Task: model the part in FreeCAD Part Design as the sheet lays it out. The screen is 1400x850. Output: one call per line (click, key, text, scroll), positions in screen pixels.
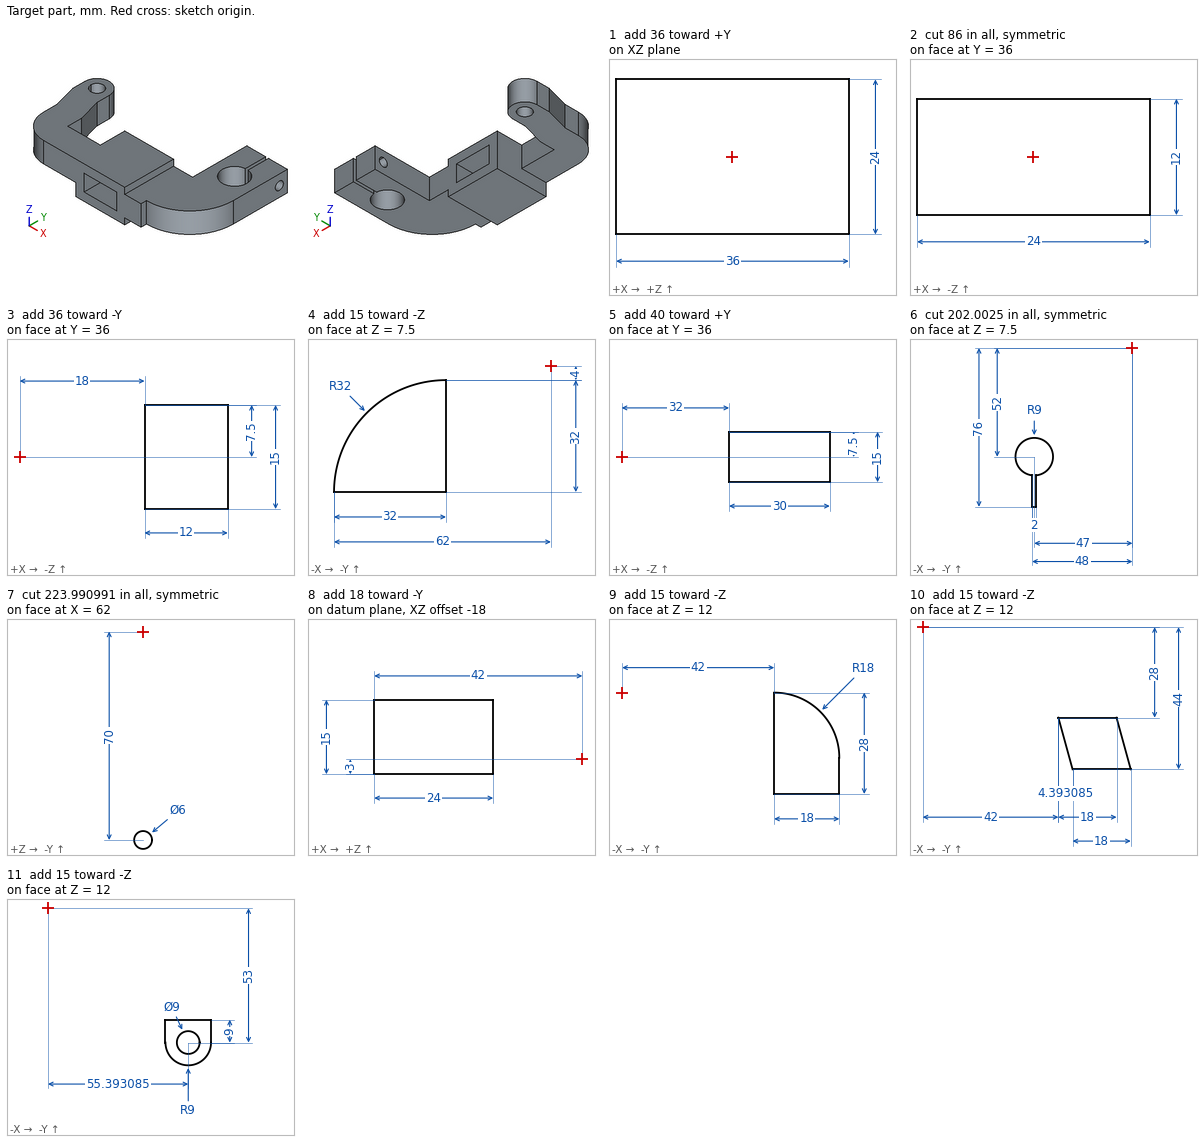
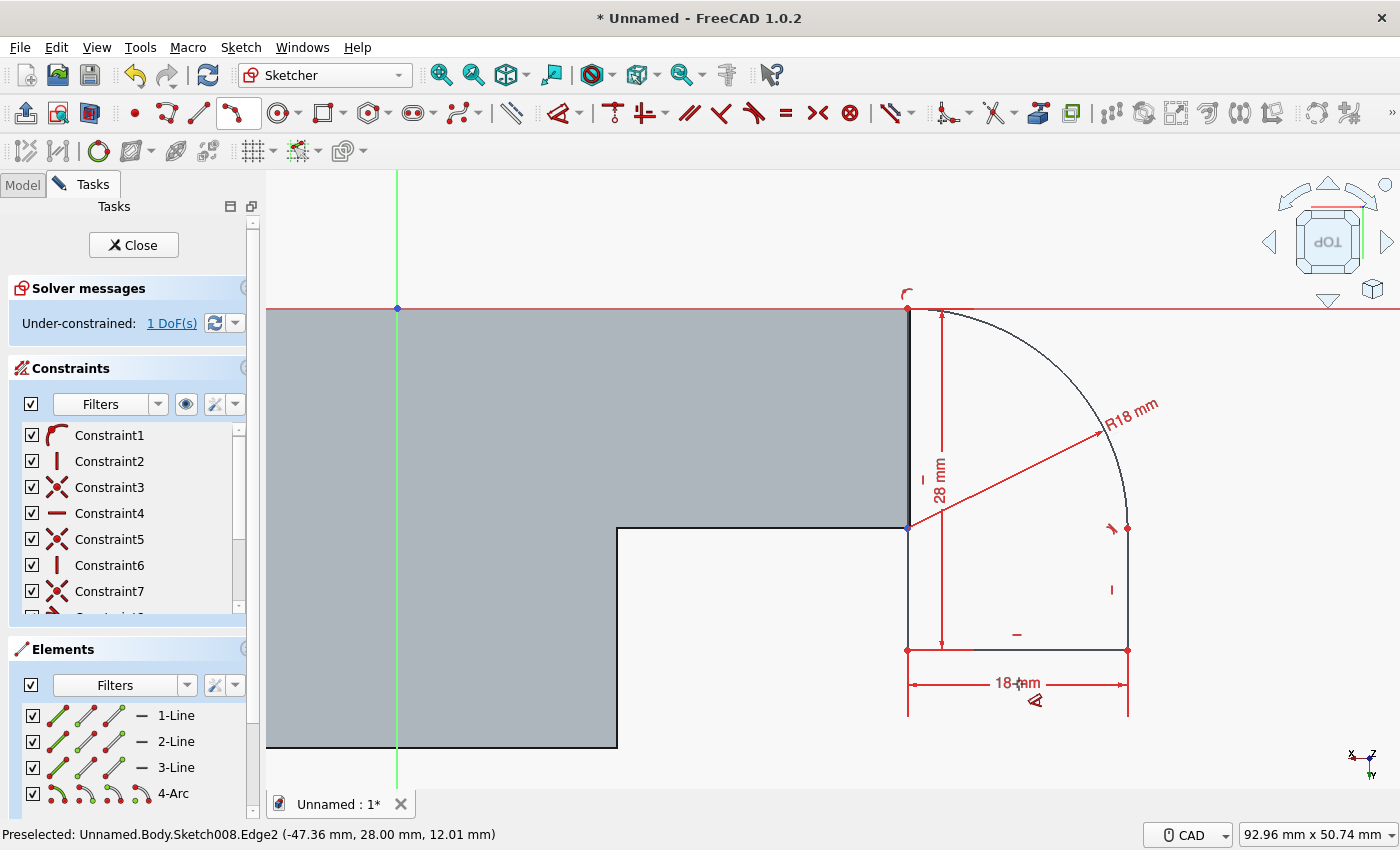
click(908, 309)
click(653, 275)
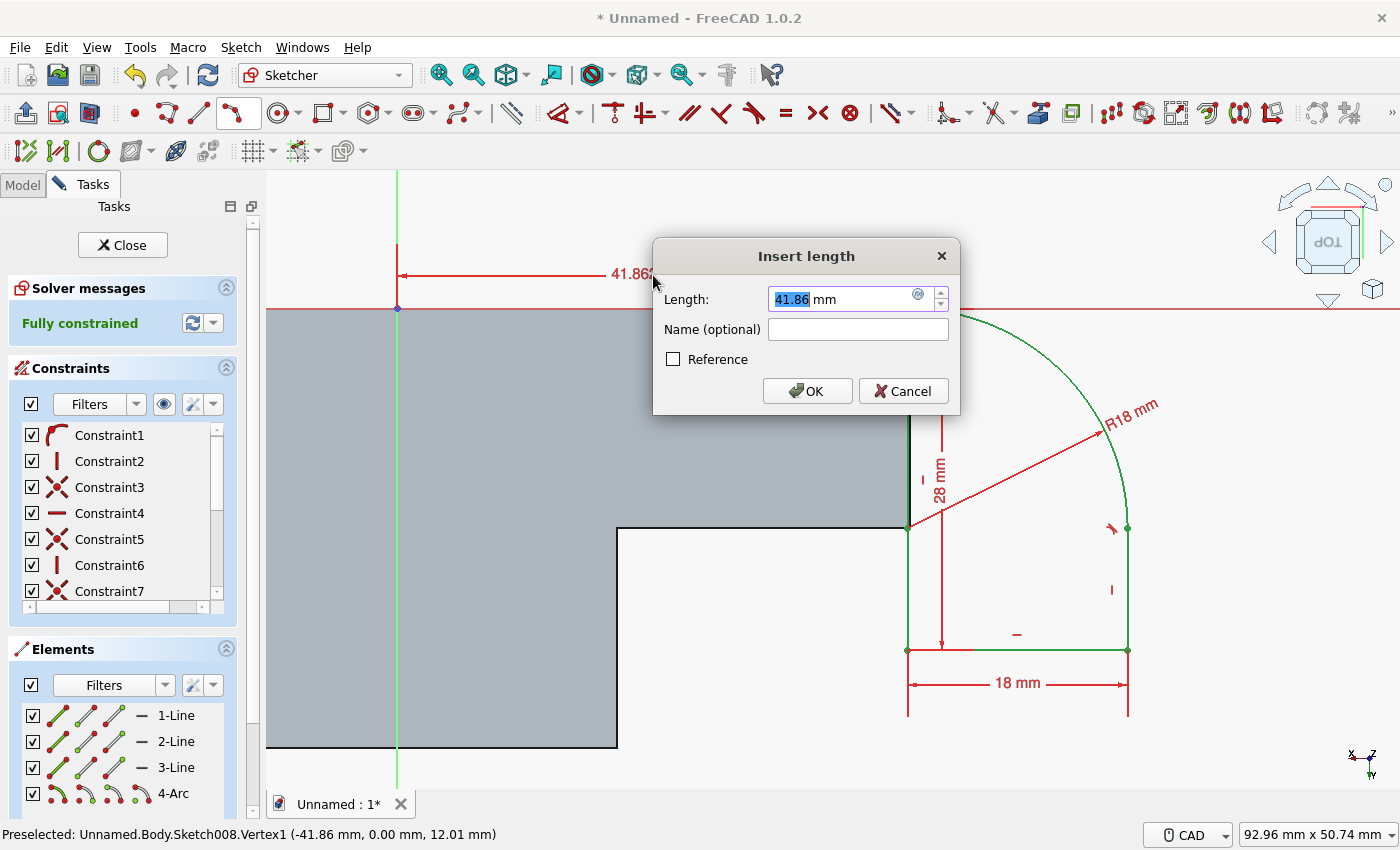
text(42)
key(Return)
key(Escape)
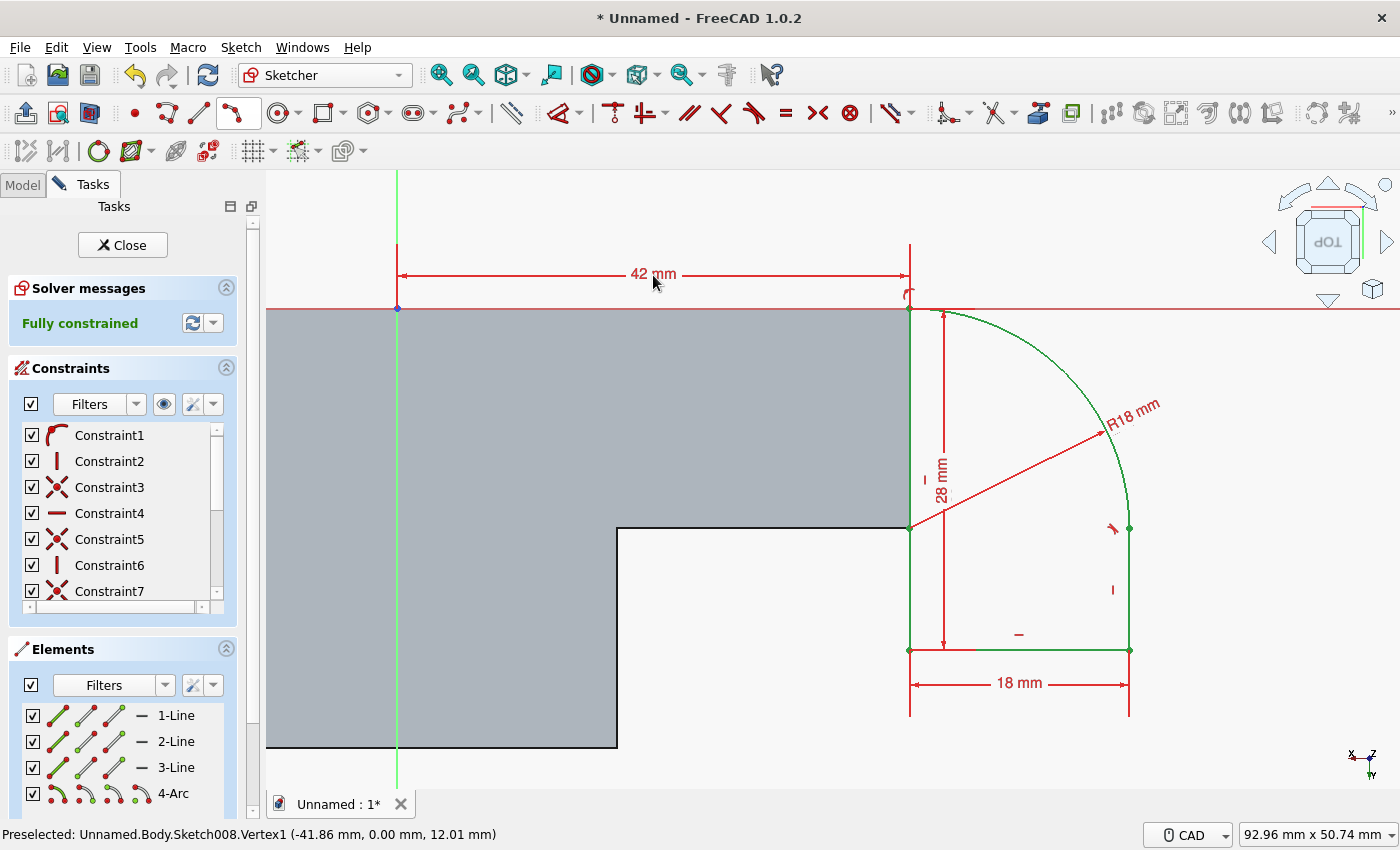
click(123, 245)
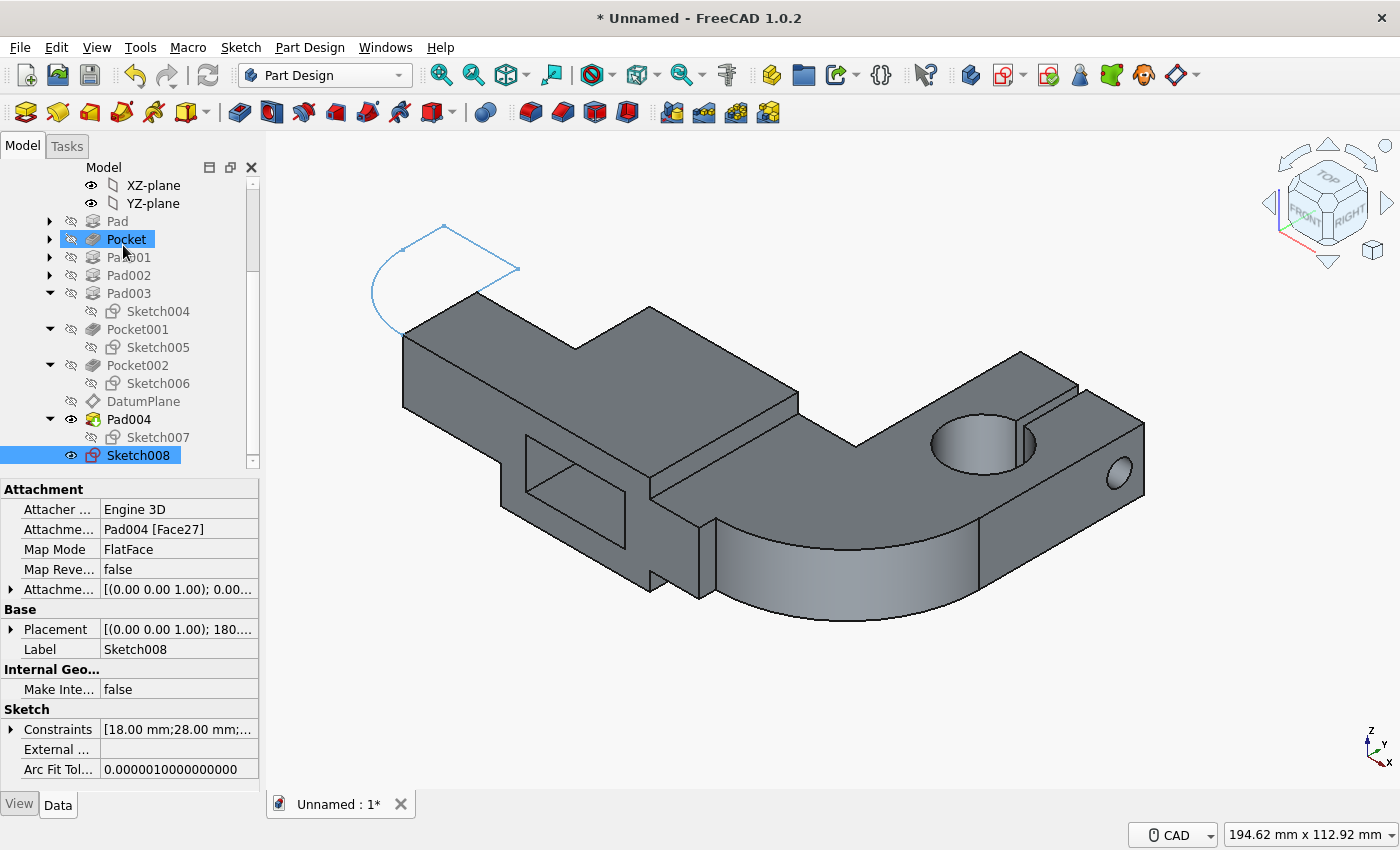
click(26, 112)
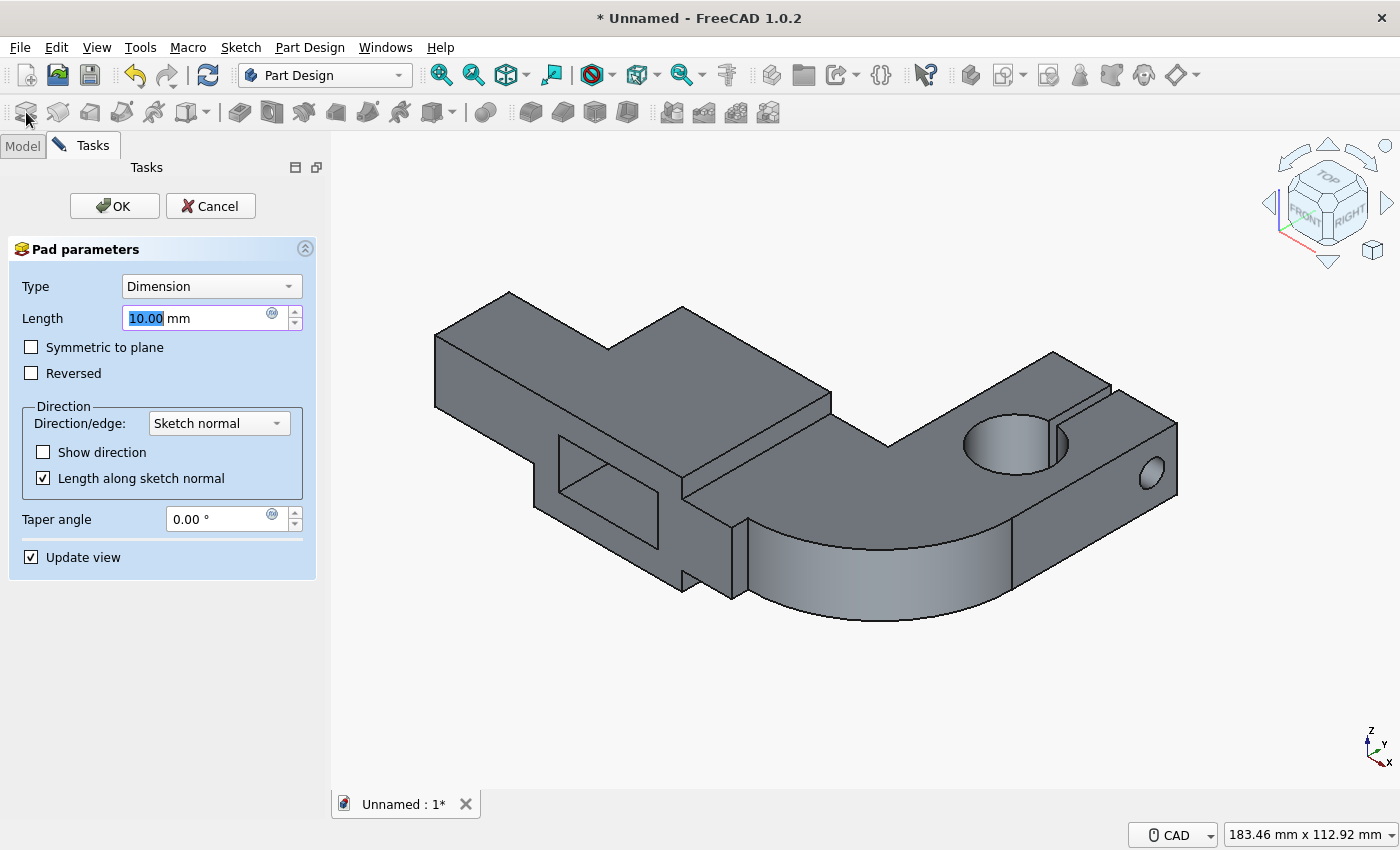
text(15)
key(Tab)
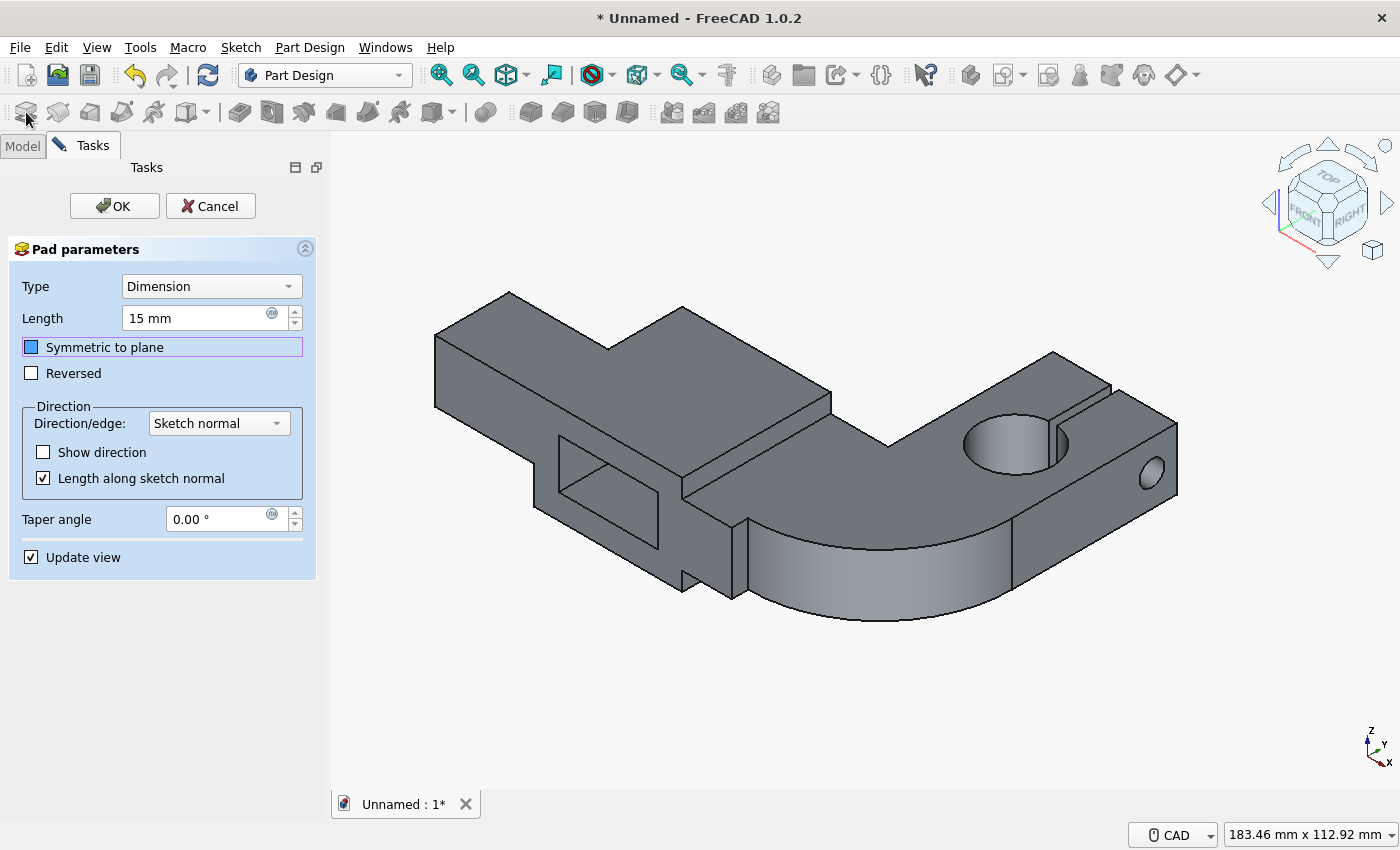
click(30, 373)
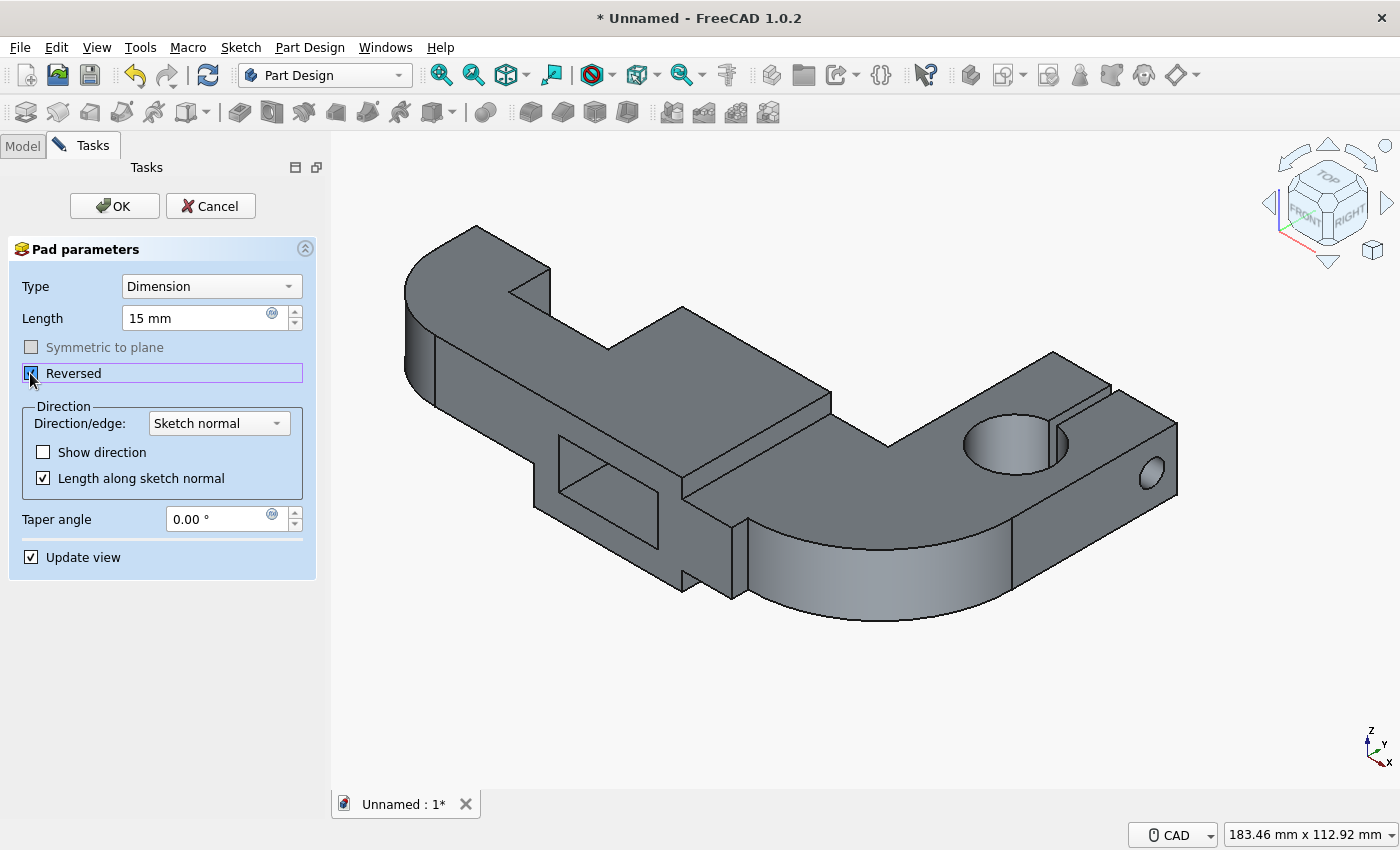
click(115, 206)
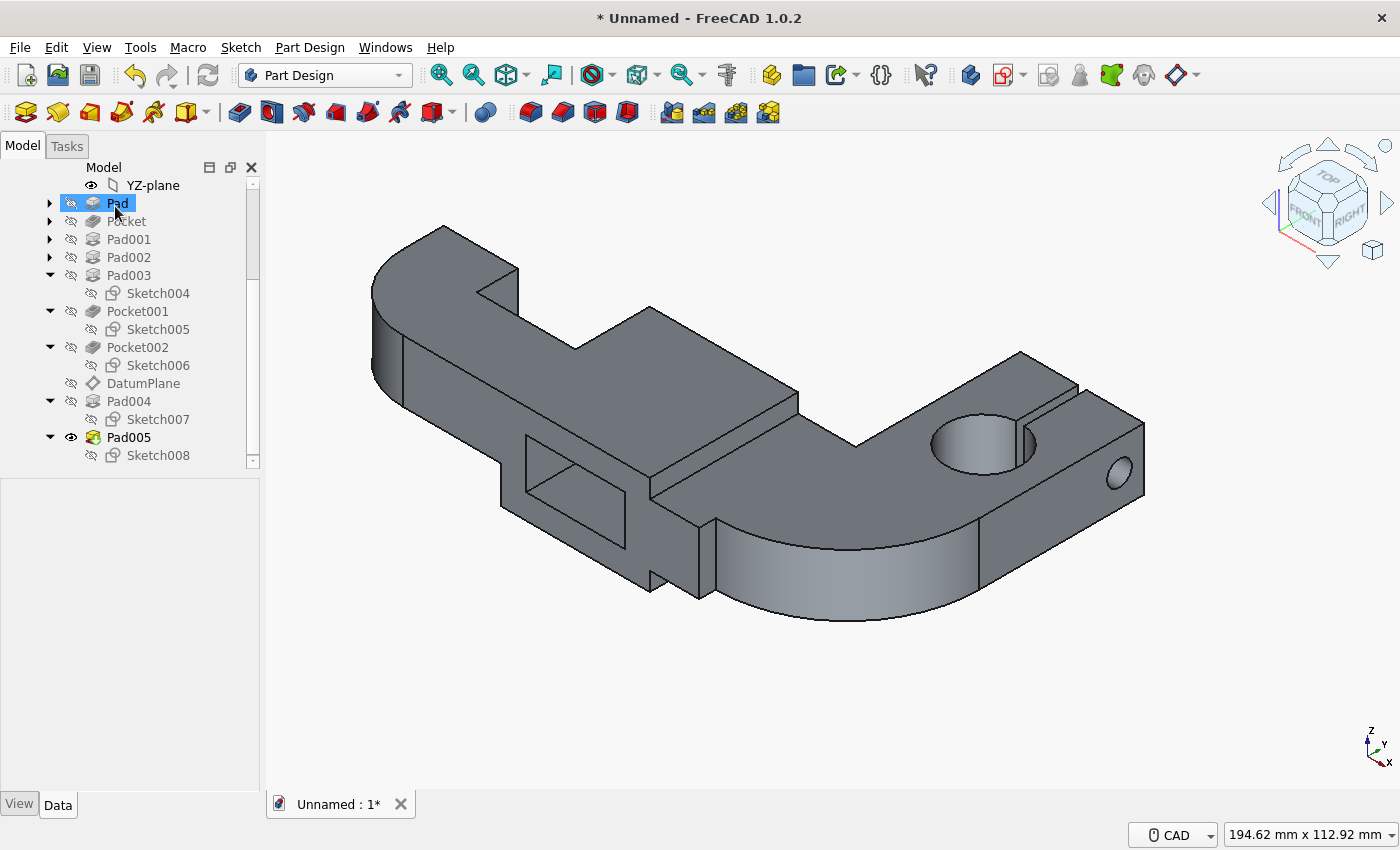
key(v)
key(f)